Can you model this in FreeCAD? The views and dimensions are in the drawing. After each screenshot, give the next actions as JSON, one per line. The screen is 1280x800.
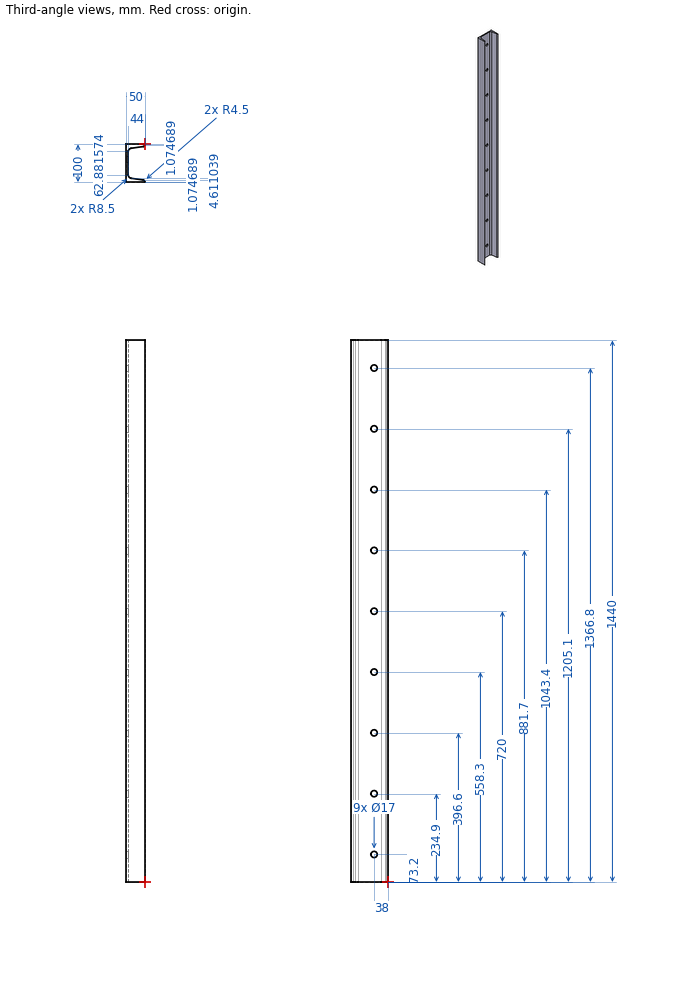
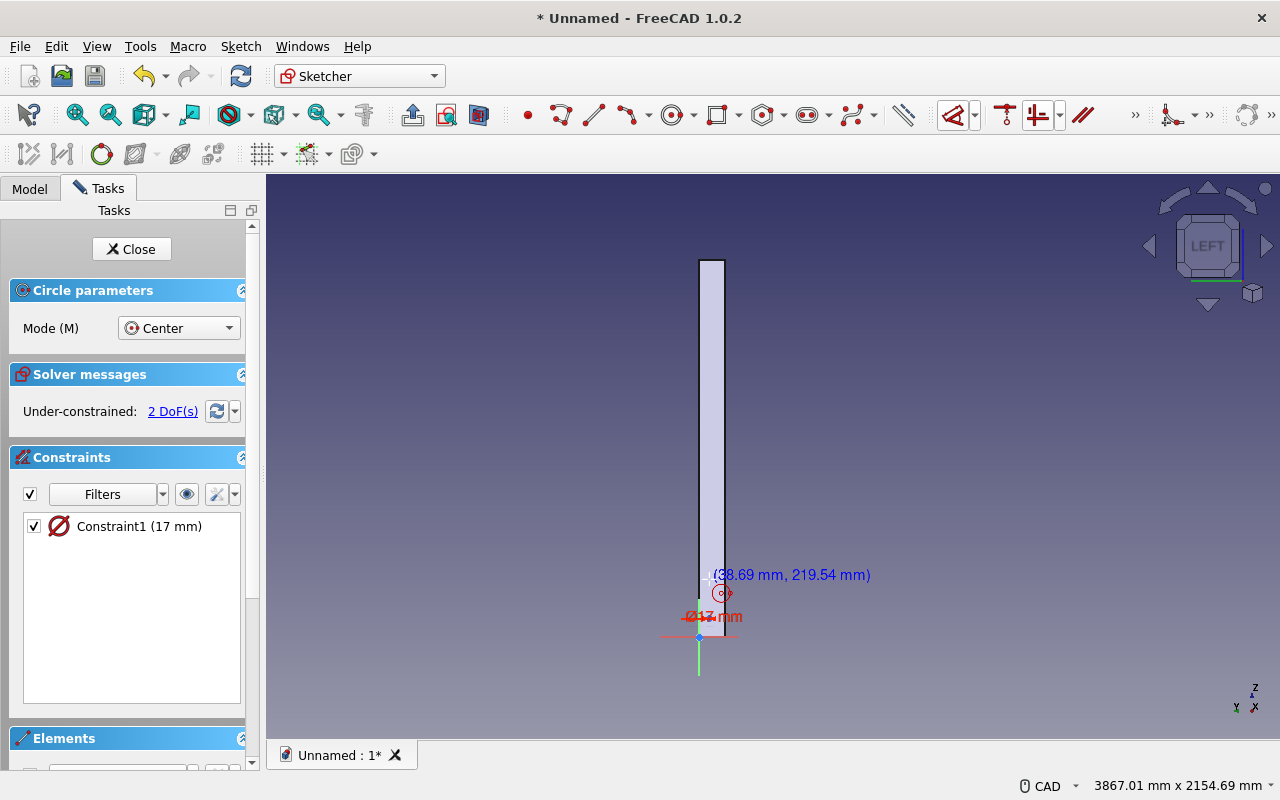
{"action": "scroll", "coordinate": [709, 576], "scroll_direction": "up", "scroll_amount": 3}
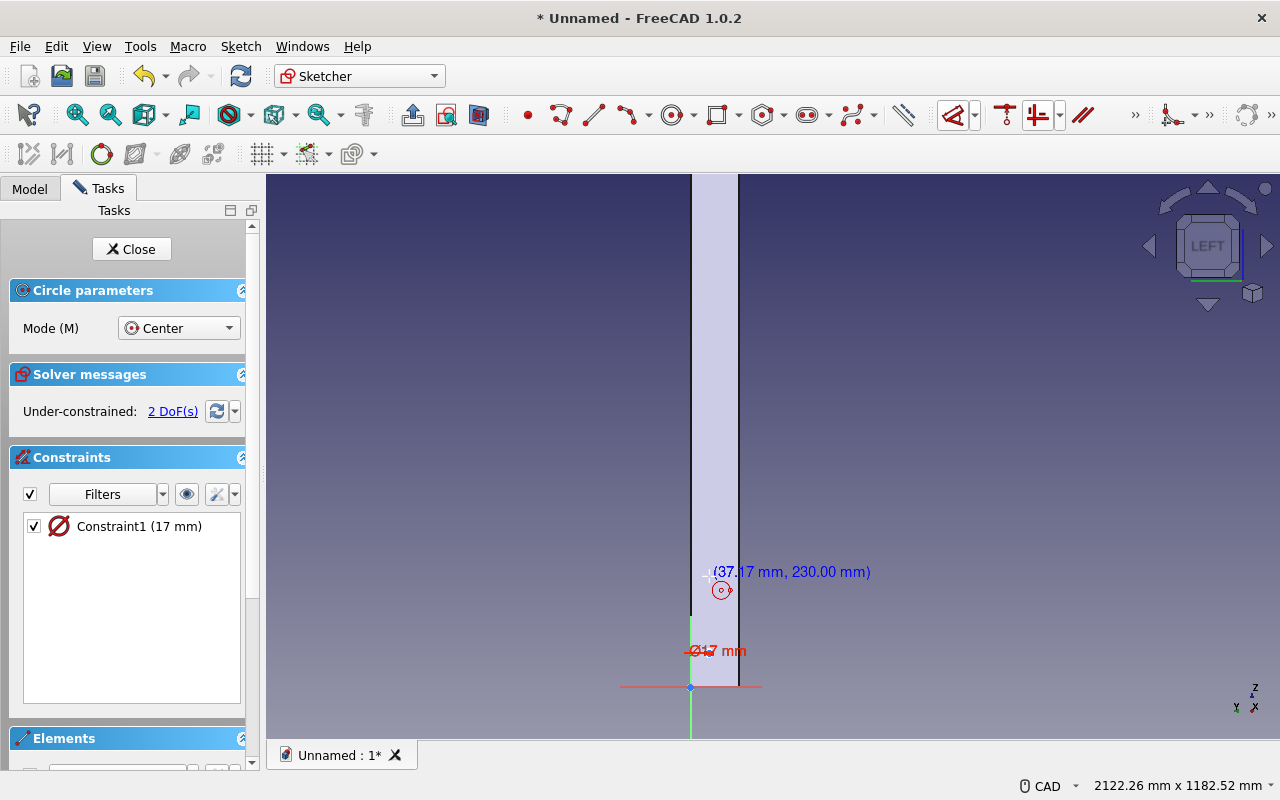
{"action": "left_click", "coordinate": [709, 575]}
{"action": "mouse_move", "coordinate": [712, 572]}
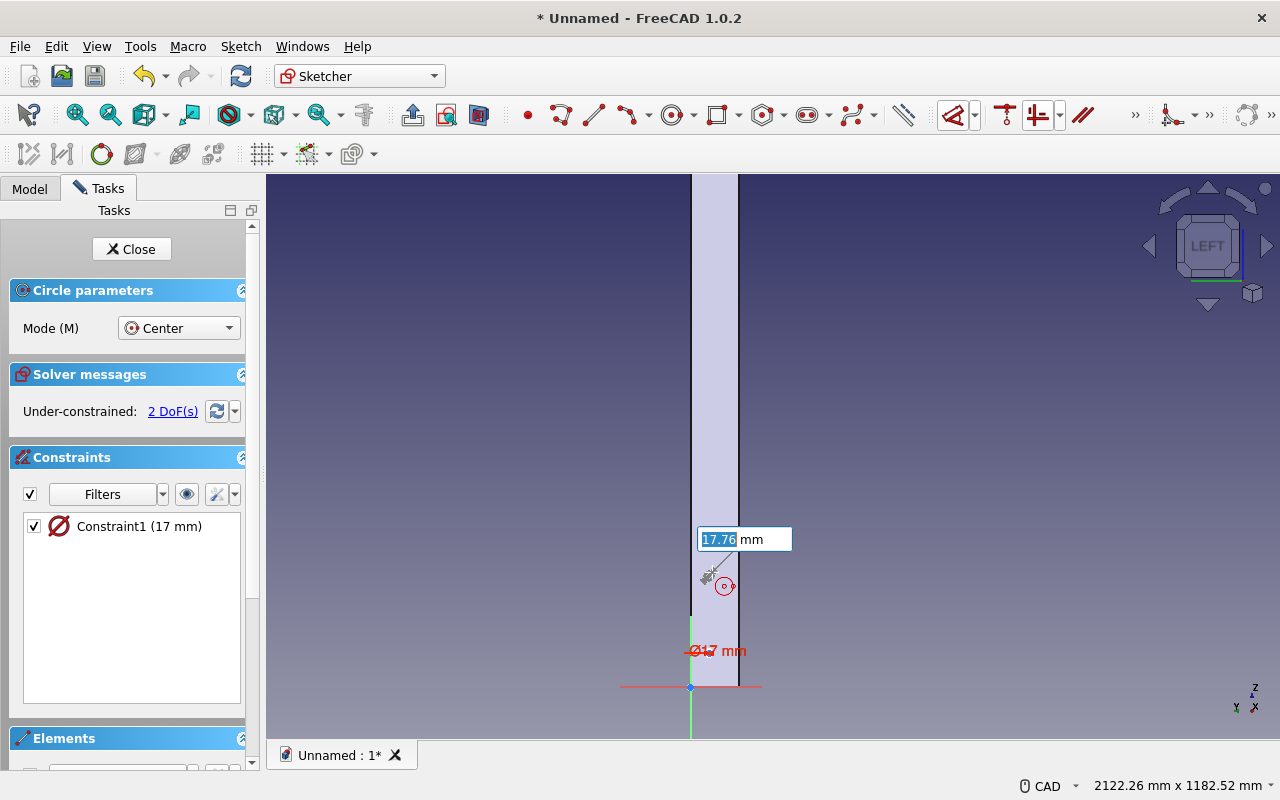
{"action": "type", "text": "17"}
{"action": "key", "text": "Return"}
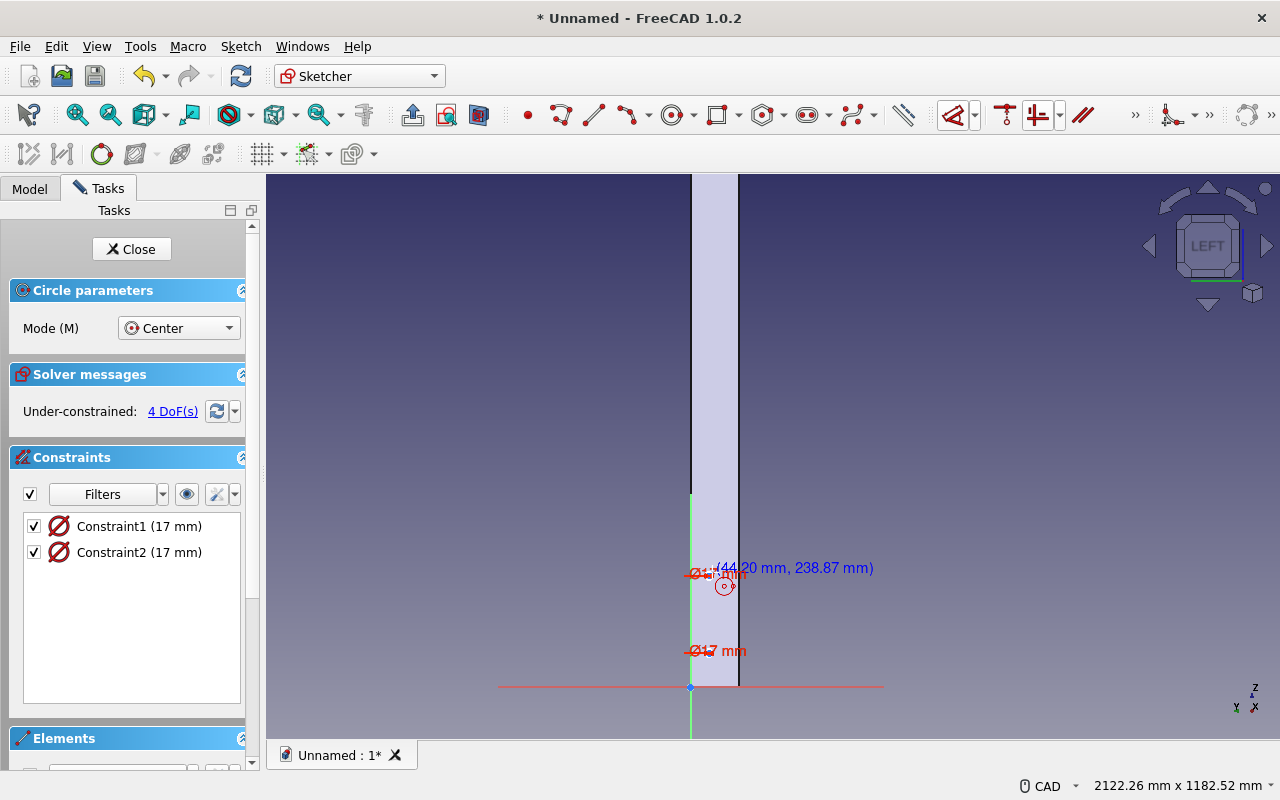
{"action": "scroll", "coordinate": [709, 498], "scroll_direction": "up", "scroll_amount": 9}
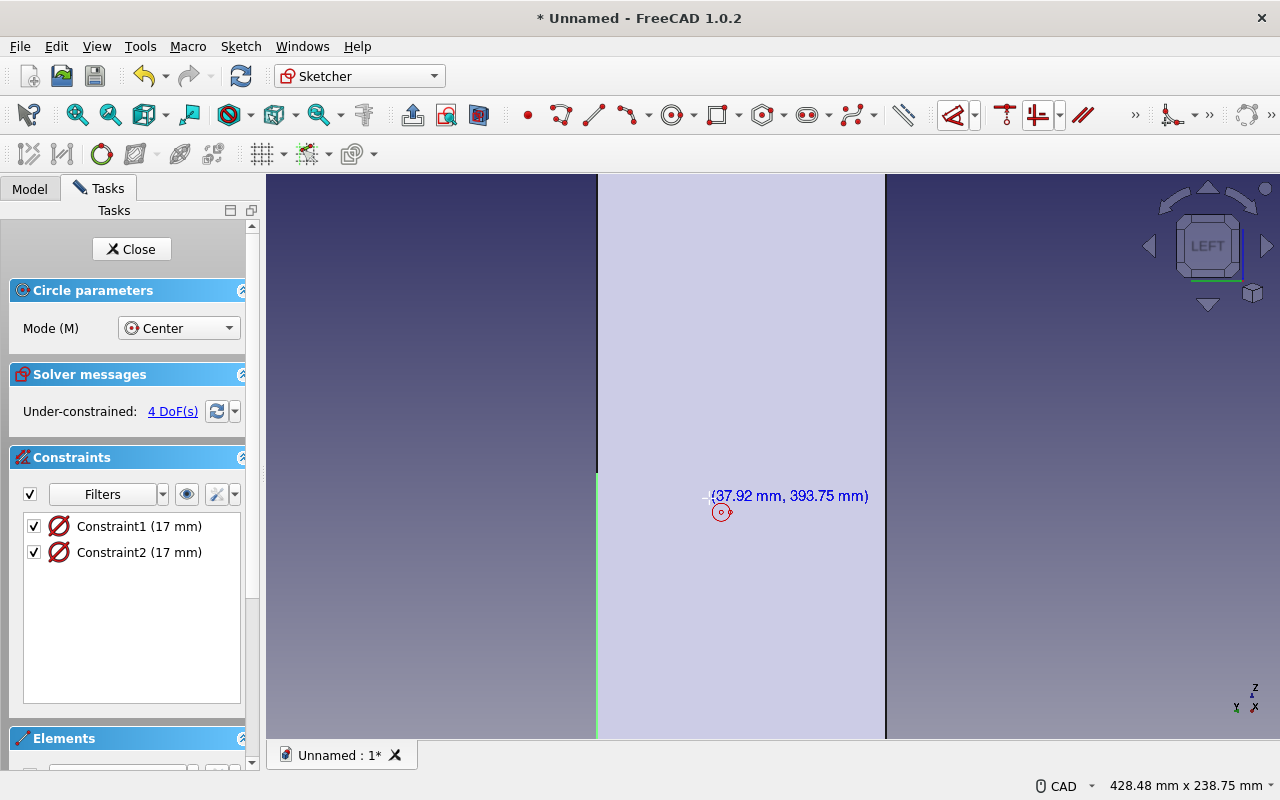
{"action": "scroll", "coordinate": [709, 537], "scroll_direction": "down", "scroll_amount": 12}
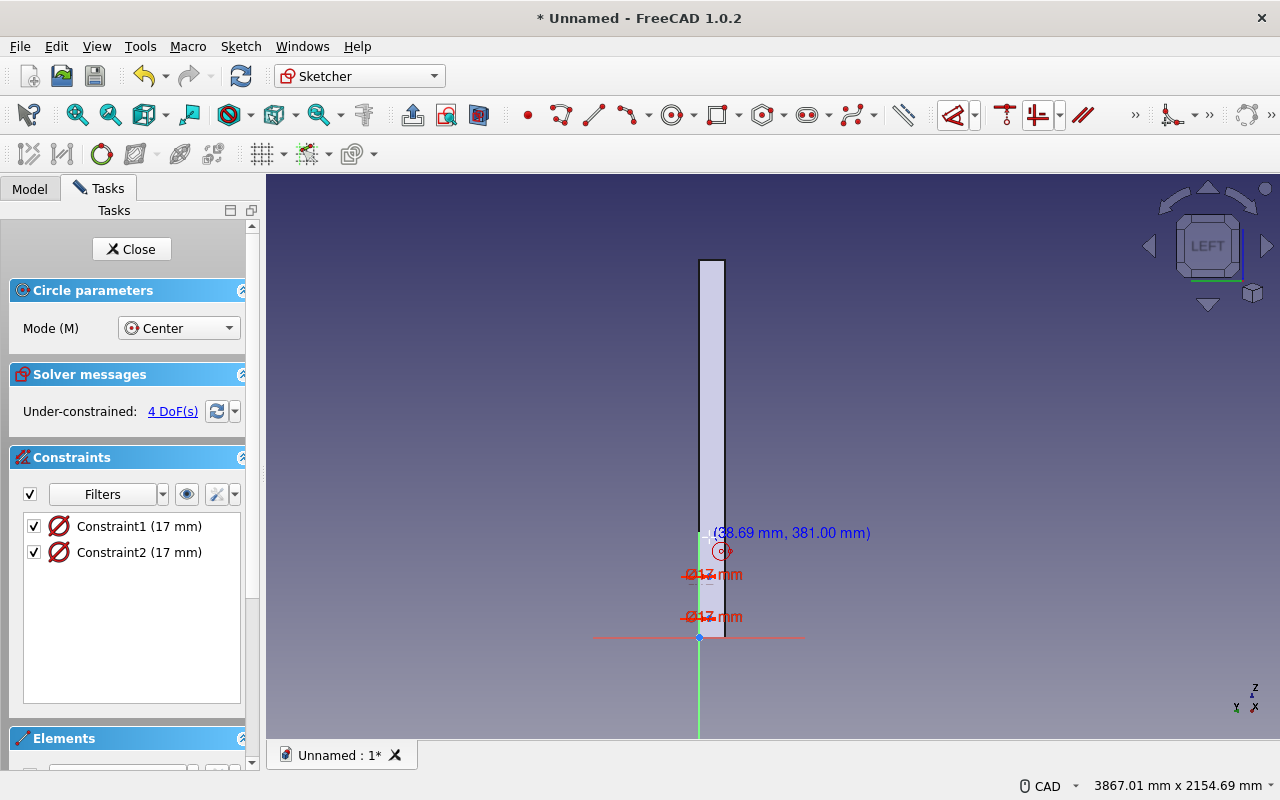
{"action": "scroll", "coordinate": [709, 534], "scroll_direction": "up", "scroll_amount": 3}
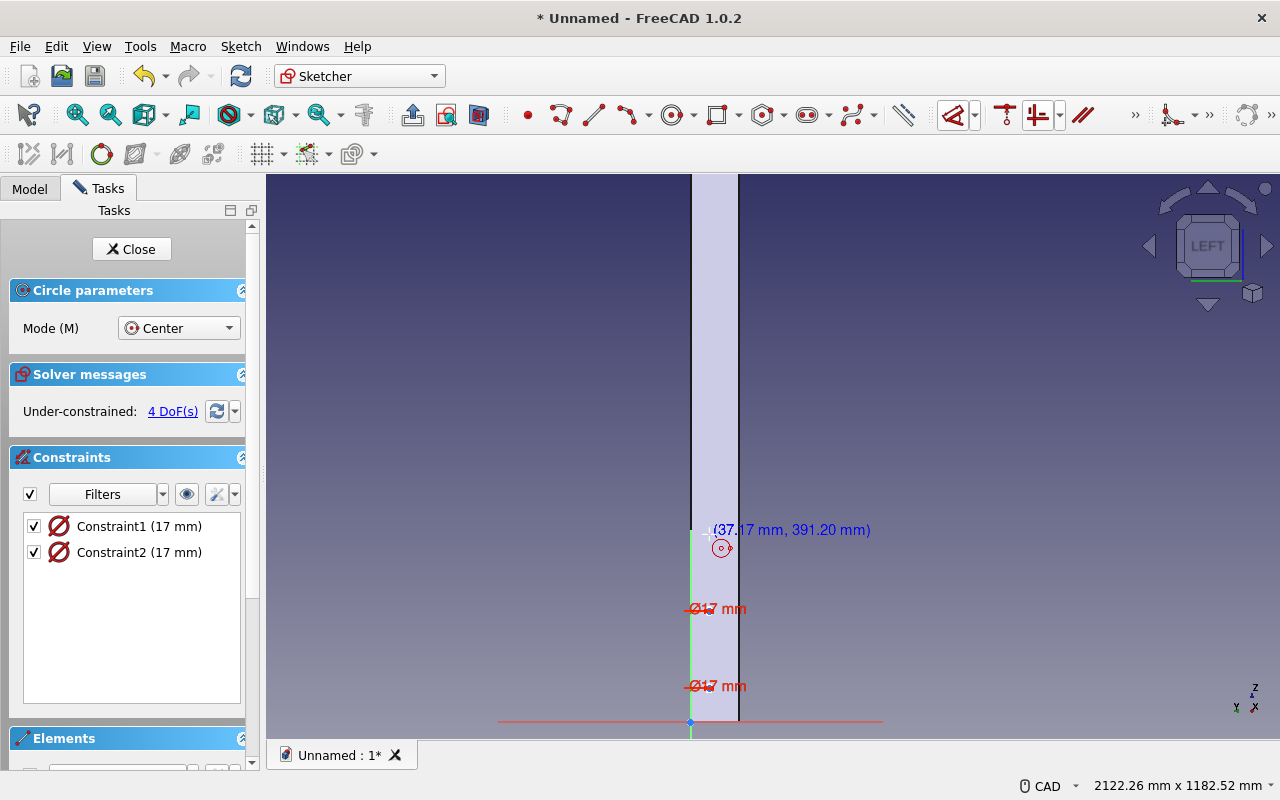
{"action": "left_click", "coordinate": [709, 533]}
{"action": "mouse_move", "coordinate": [712, 530]}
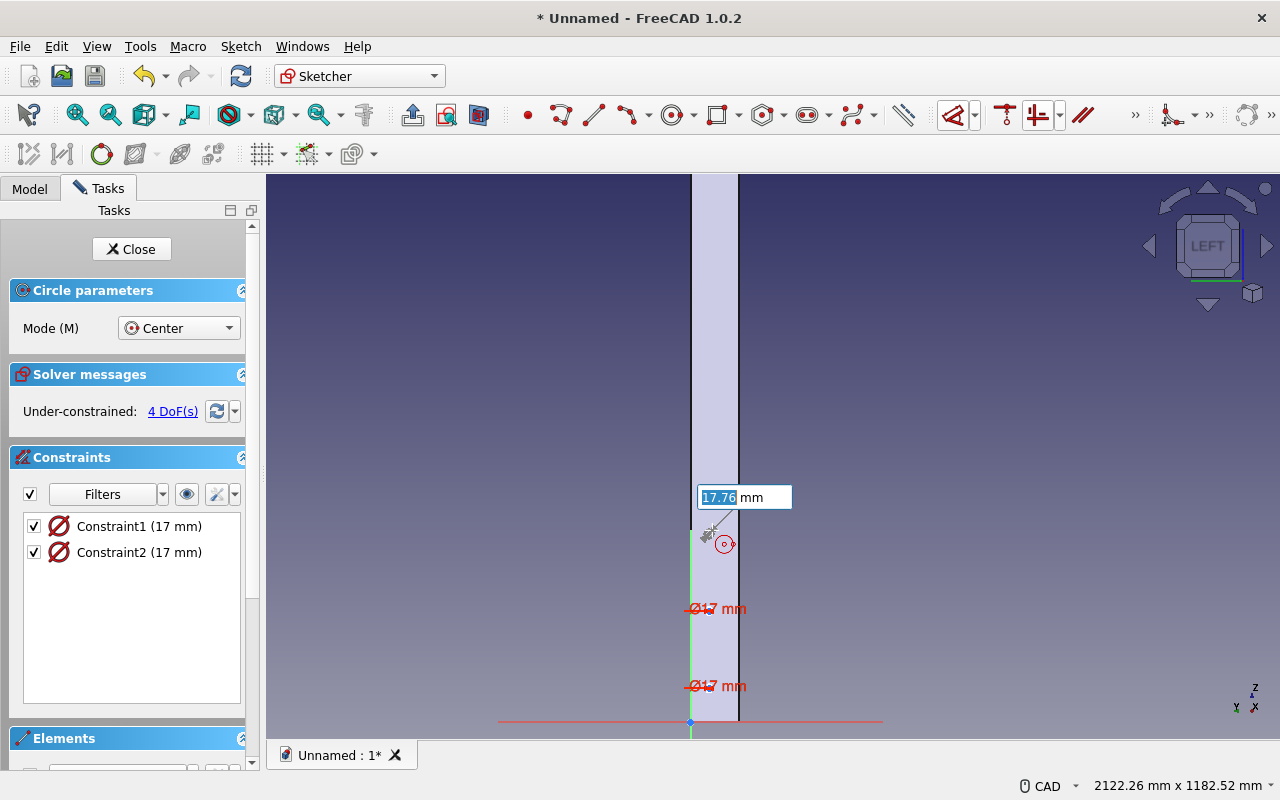
{"action": "type", "text": "17"}
{"action": "key", "text": "Return"}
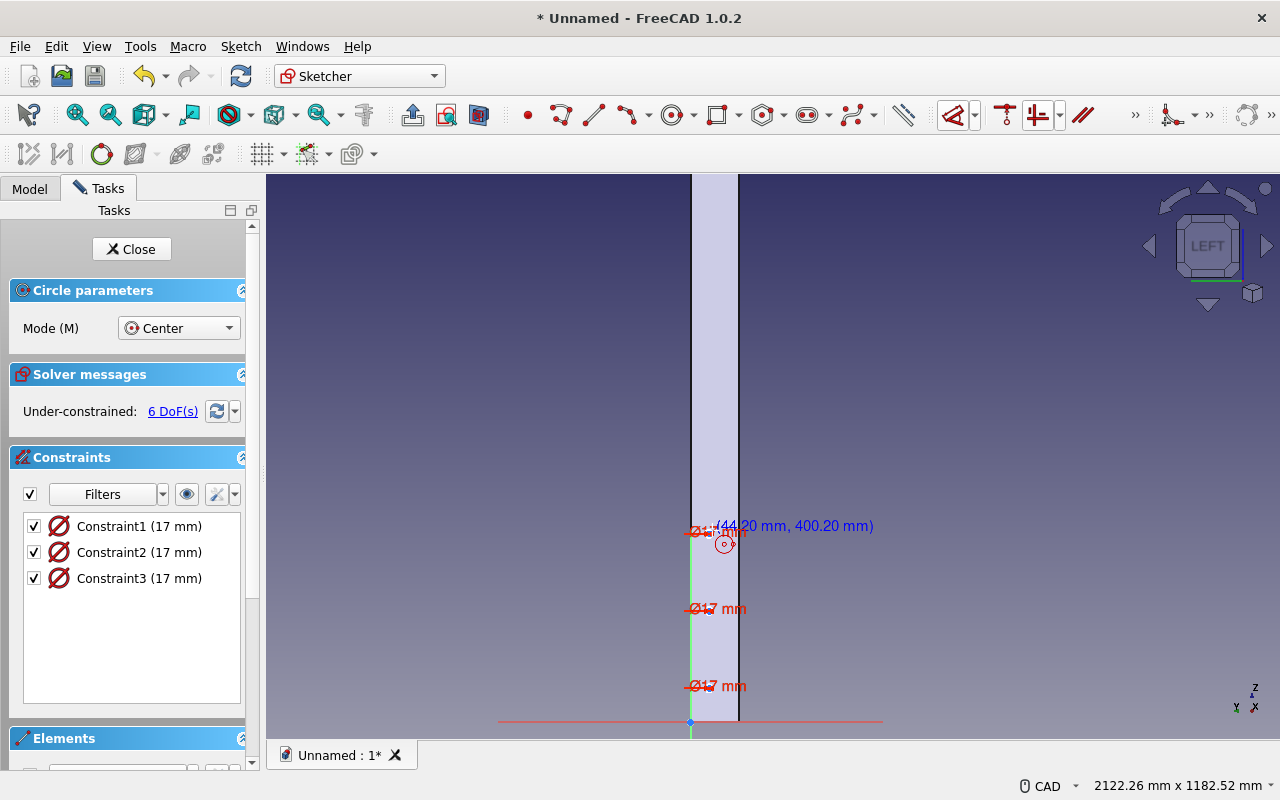
{"action": "scroll", "coordinate": [709, 455], "scroll_direction": "up", "scroll_amount": 9}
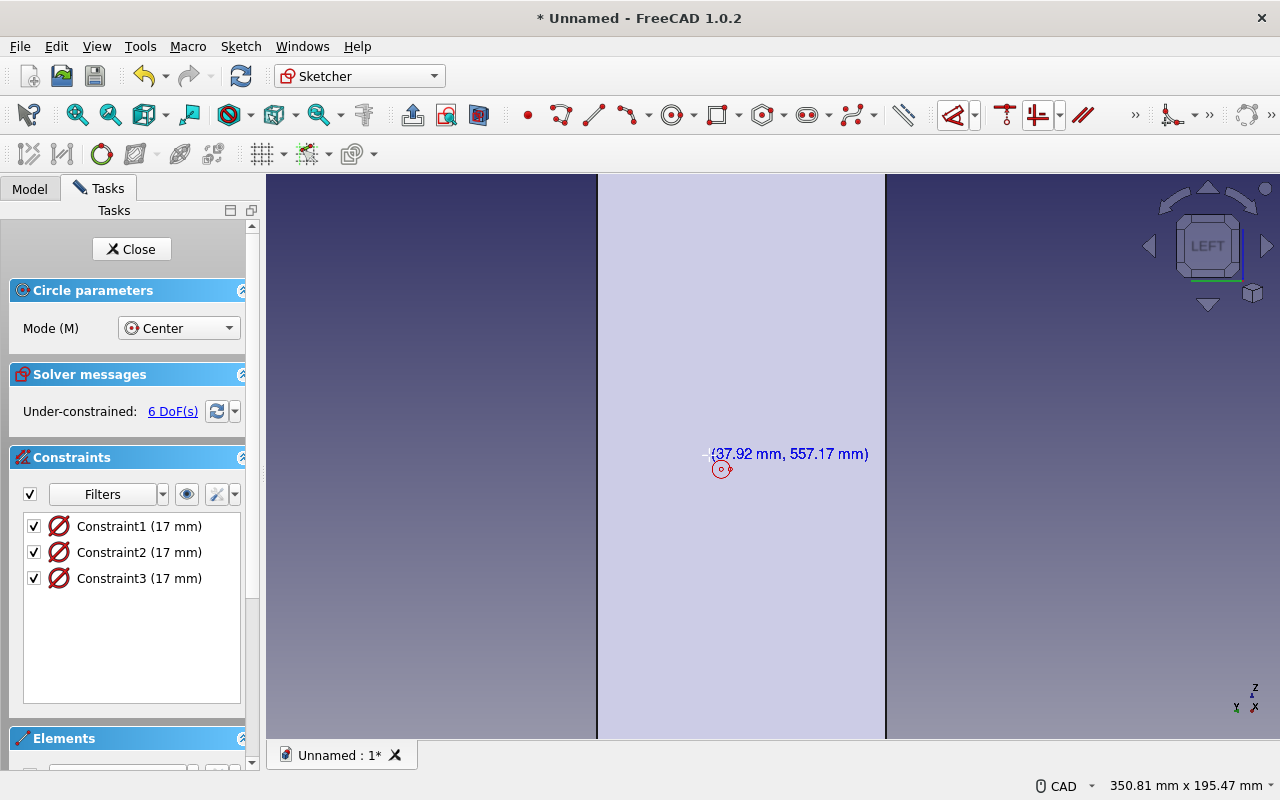
{"action": "scroll", "coordinate": [709, 494], "scroll_direction": "down", "scroll_amount": 12}